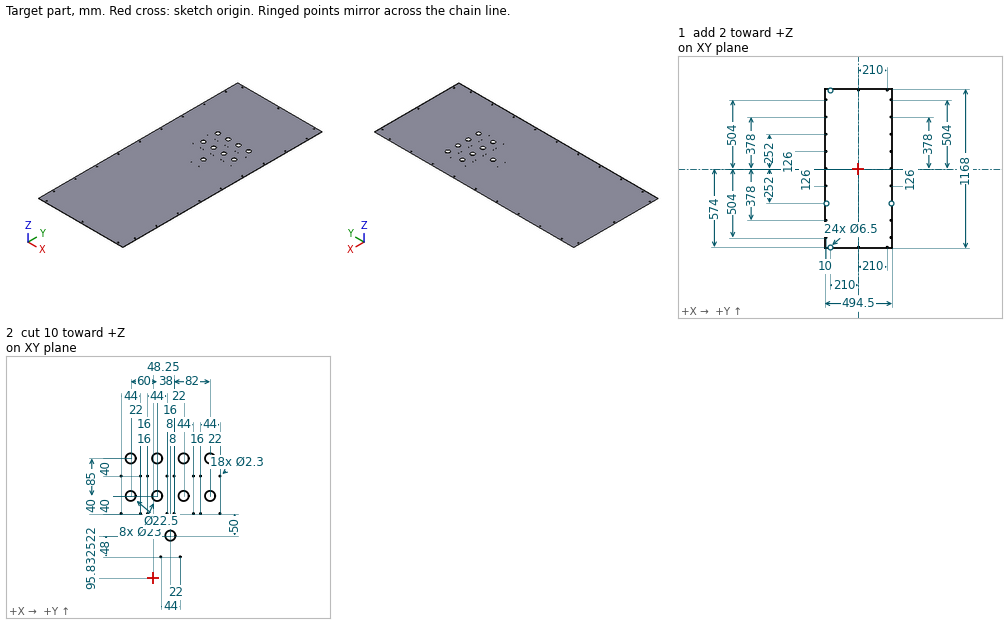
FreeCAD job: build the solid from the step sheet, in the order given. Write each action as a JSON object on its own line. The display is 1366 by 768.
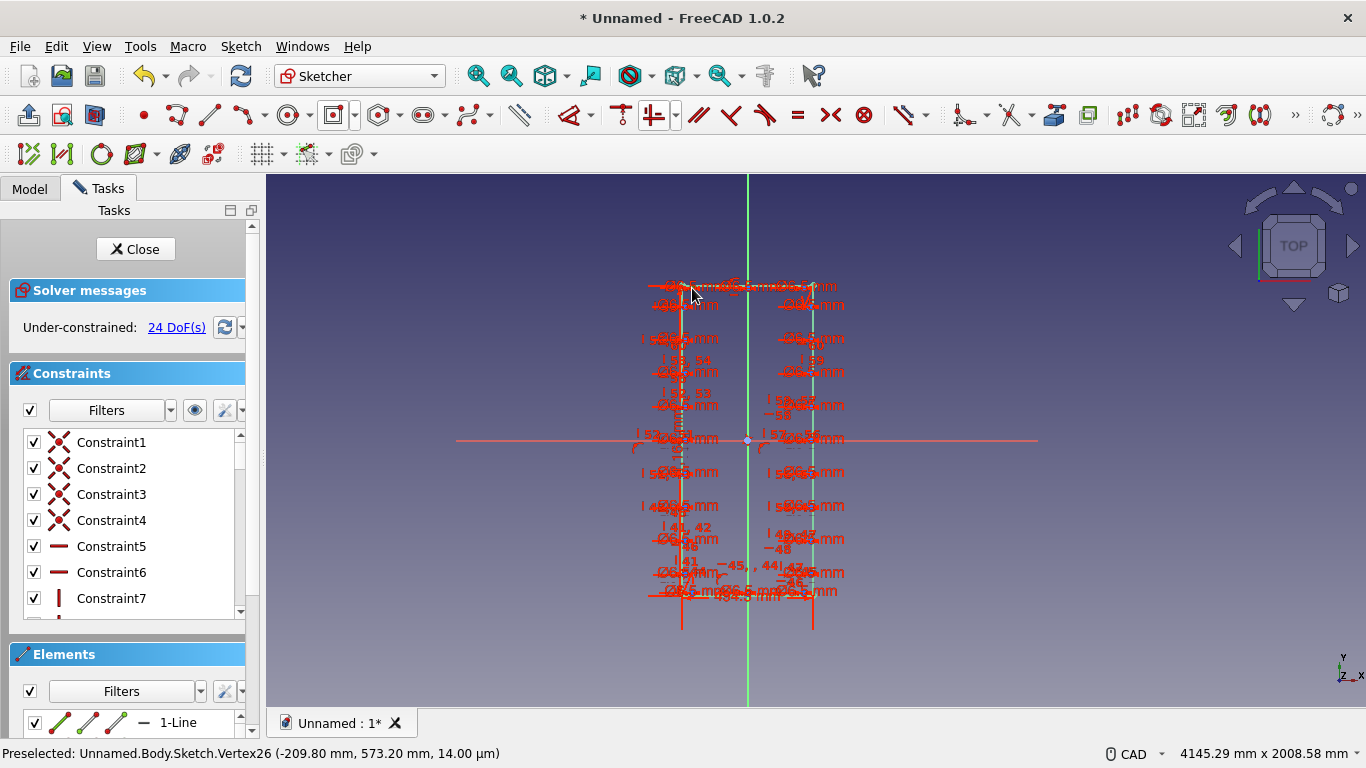
{"action": "left_click", "coordinate": [748, 288]}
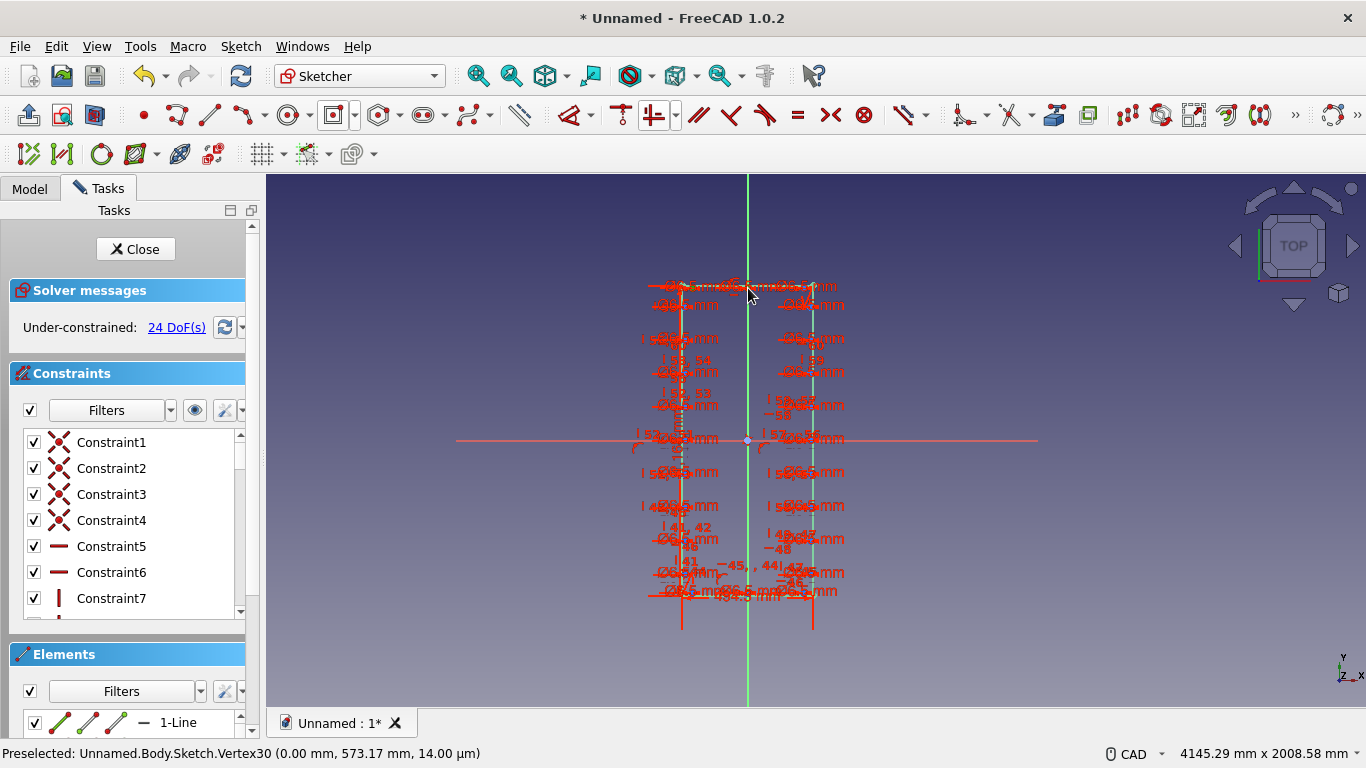
{"action": "left_click", "coordinate": [676, 116]}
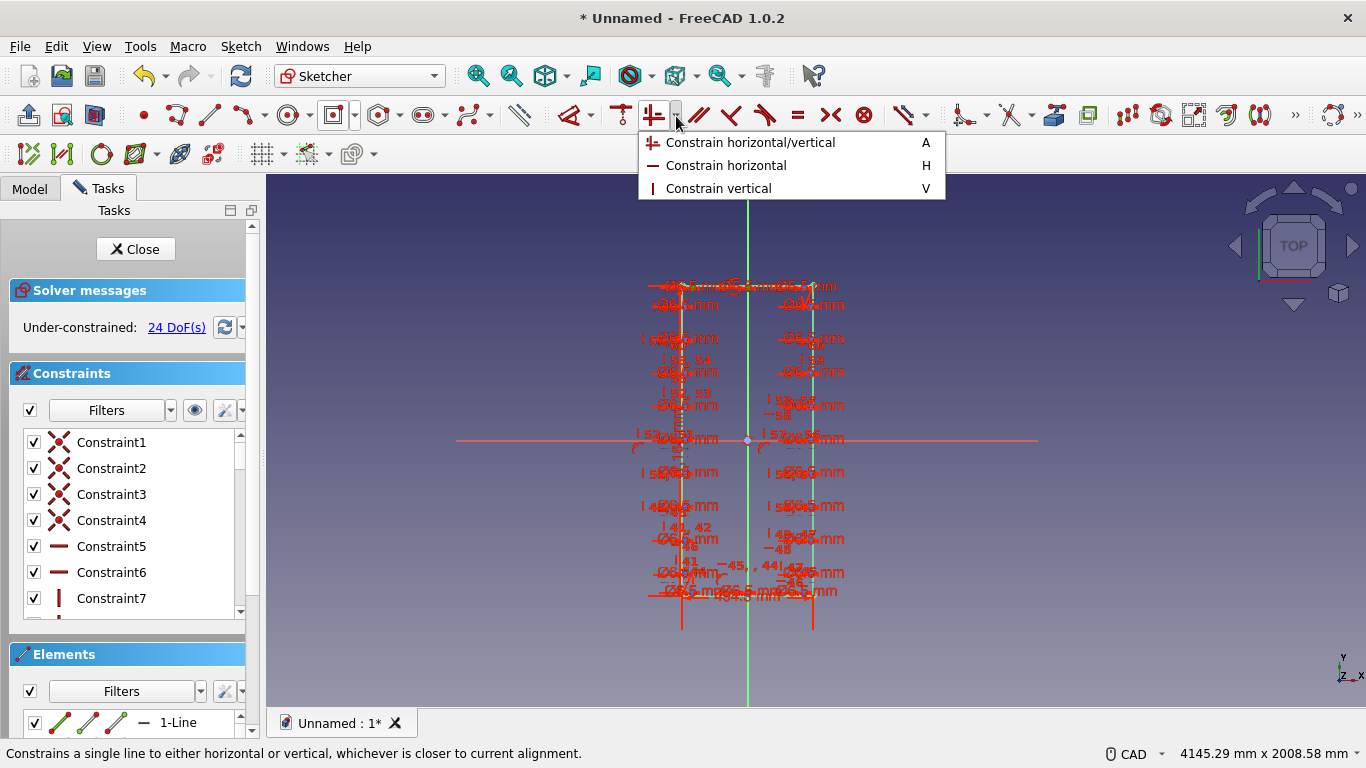
{"action": "left_click", "coordinate": [792, 166]}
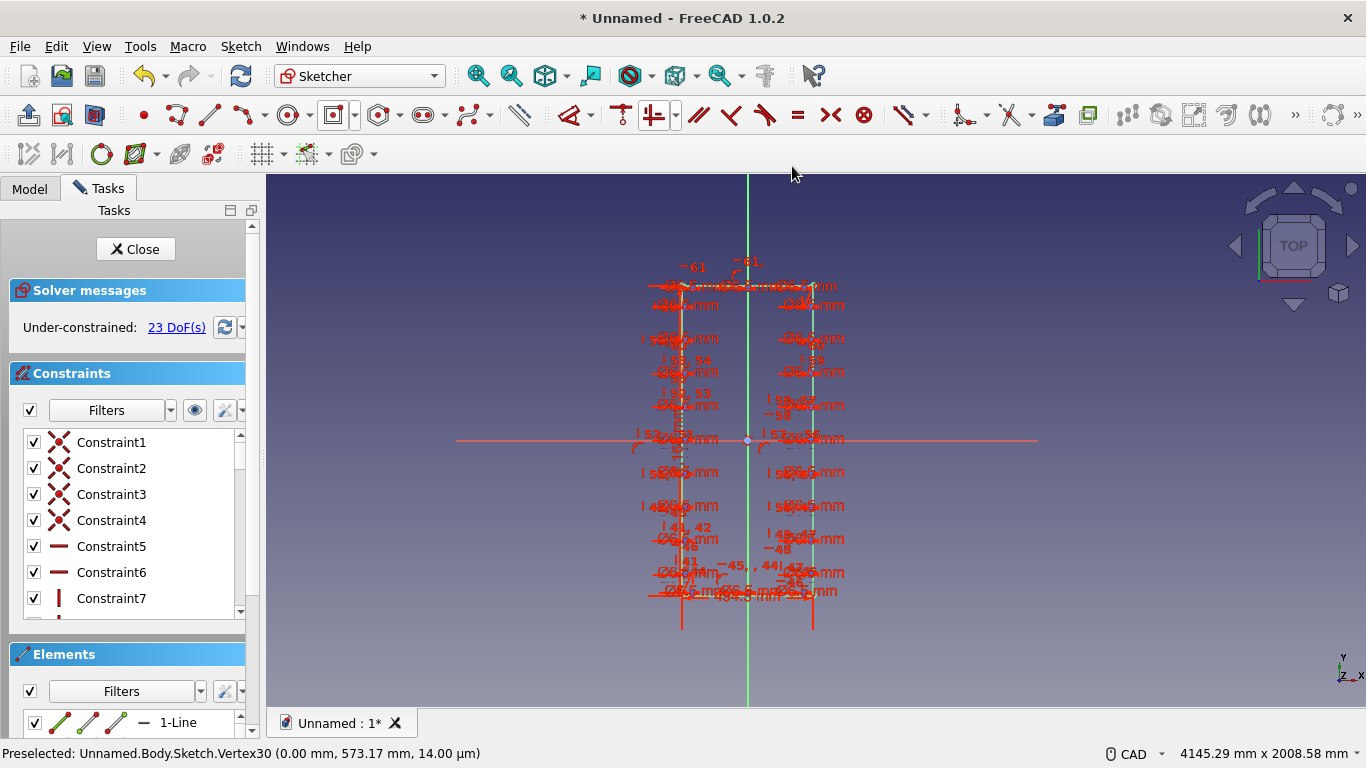
{"action": "left_click", "coordinate": [811, 374]}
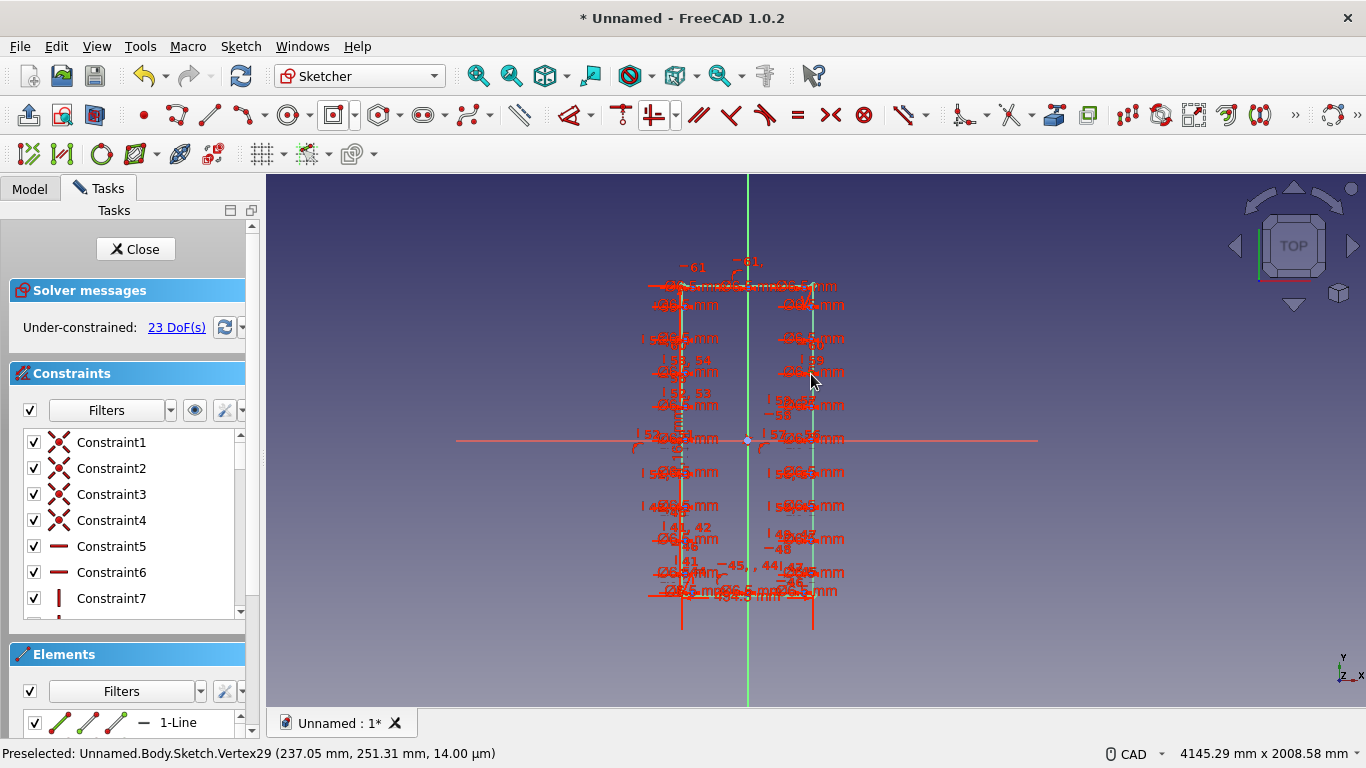
{"action": "scroll", "coordinate": [811, 340], "scroll_direction": "up", "scroll_amount": 4}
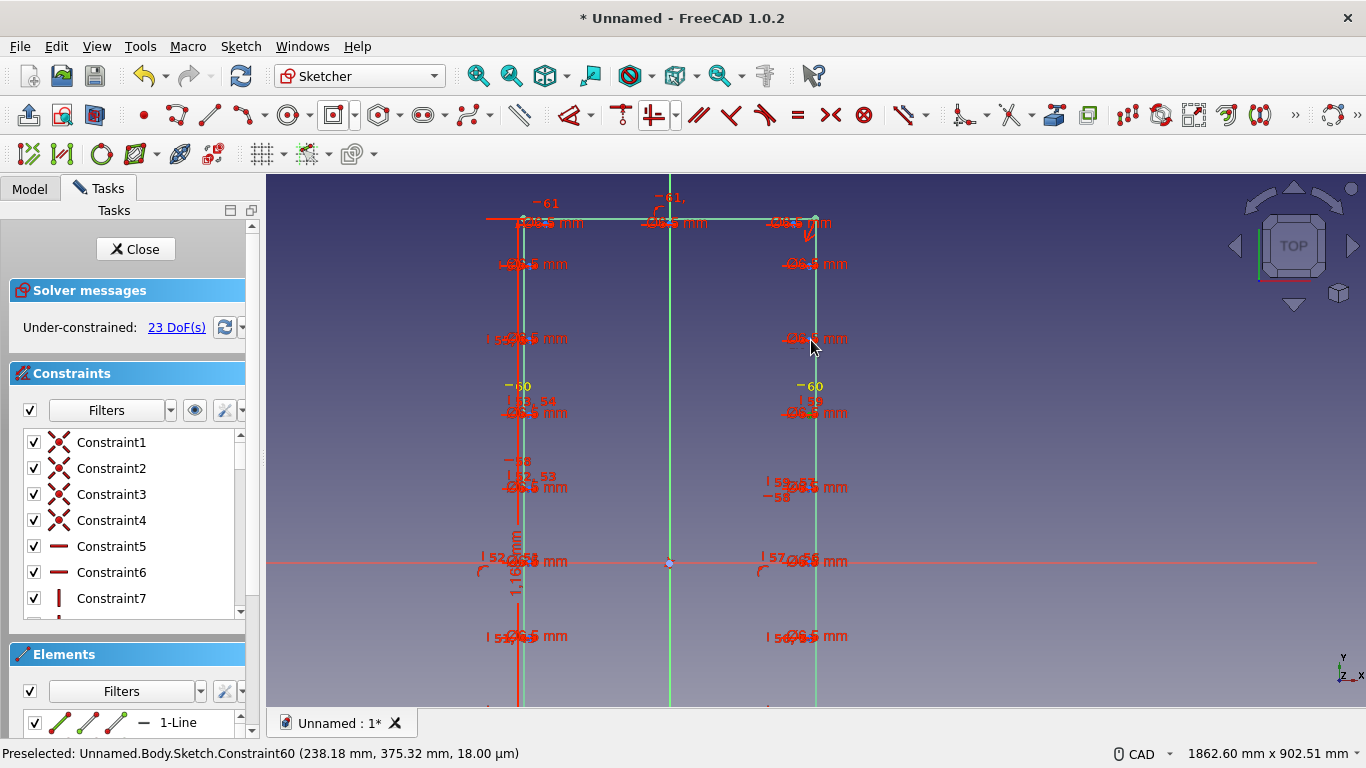
{"action": "left_click", "coordinate": [810, 341]}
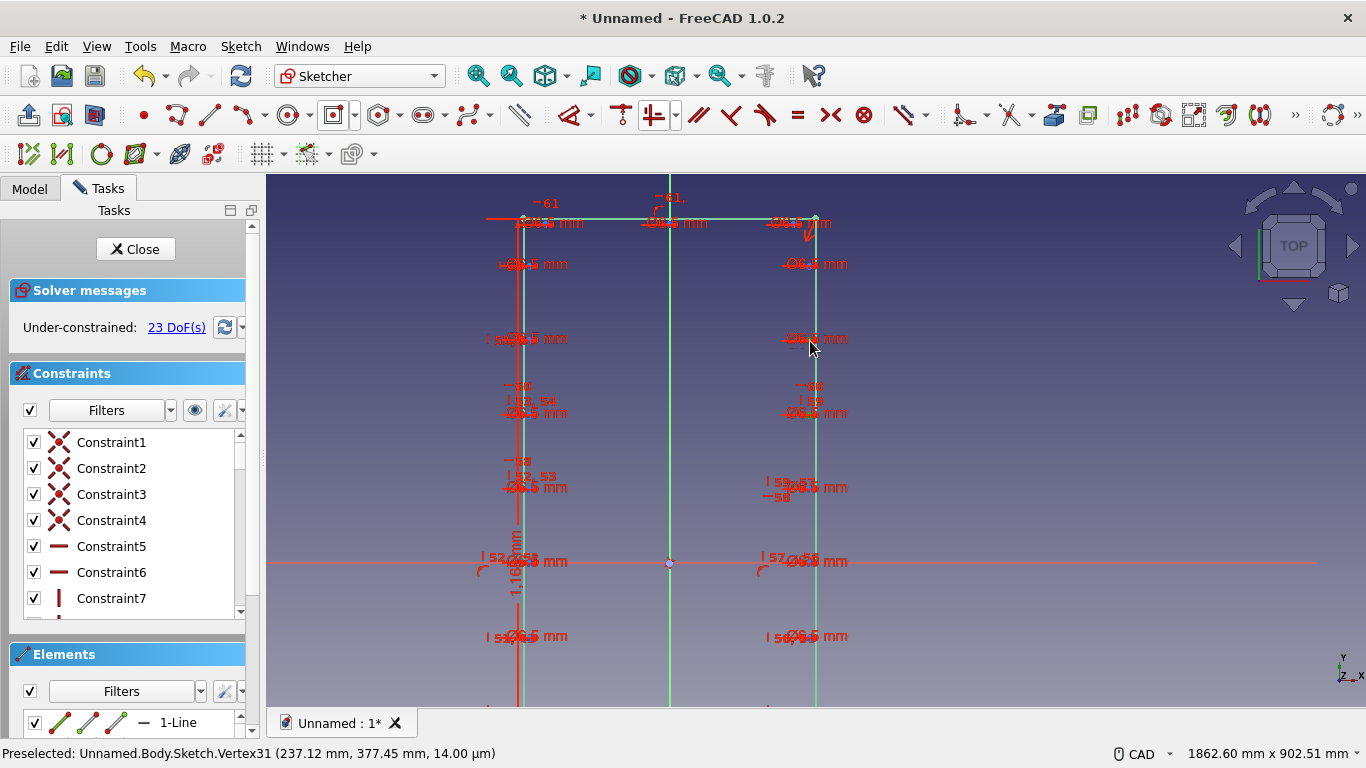
{"action": "left_click", "coordinate": [676, 116]}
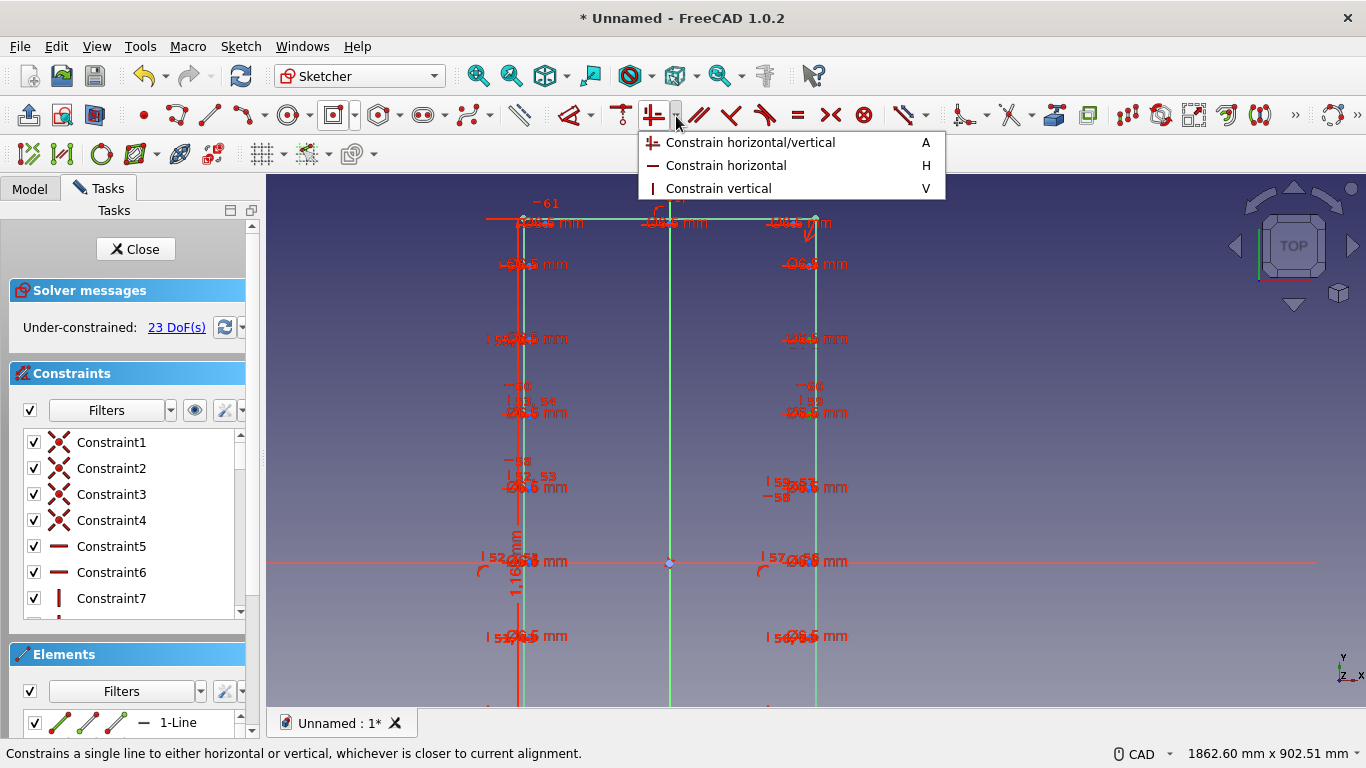
{"action": "left_click", "coordinate": [792, 188]}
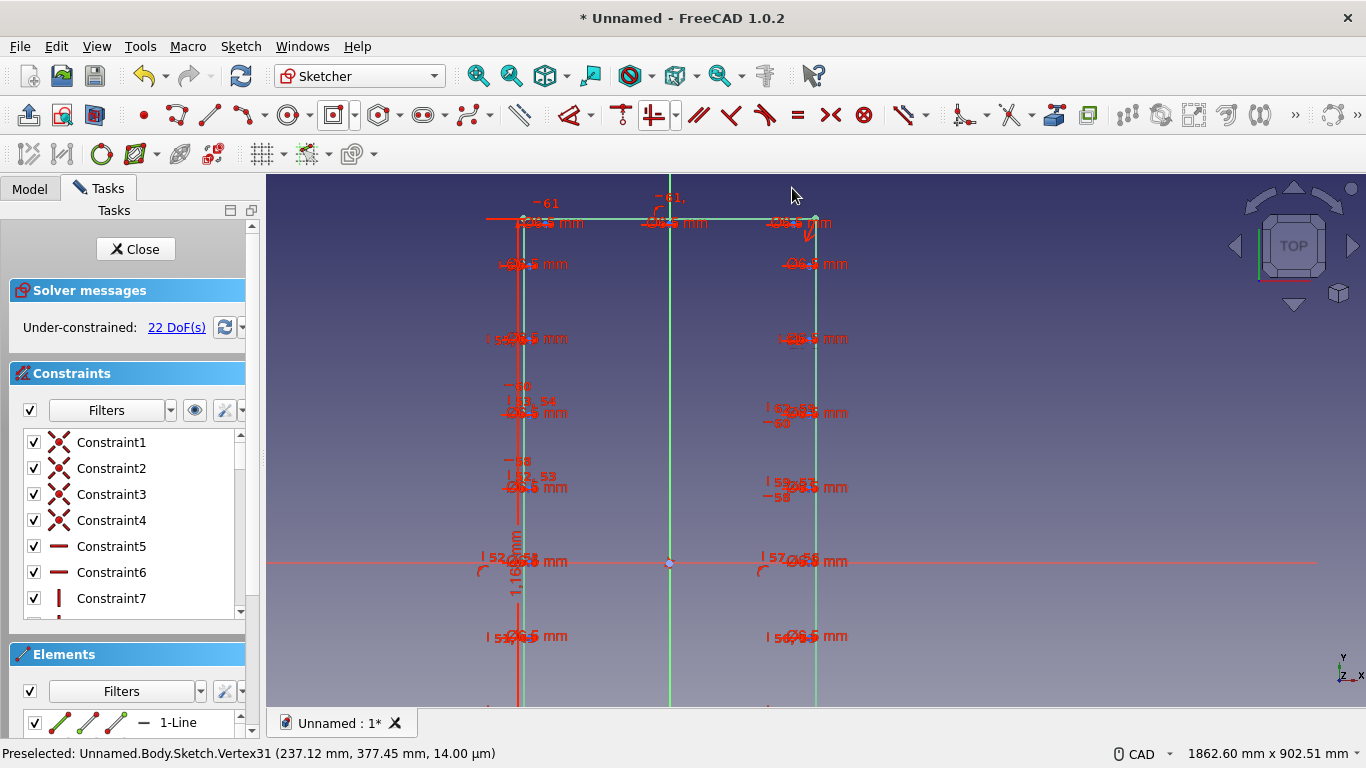
{"action": "left_click", "coordinate": [810, 341]}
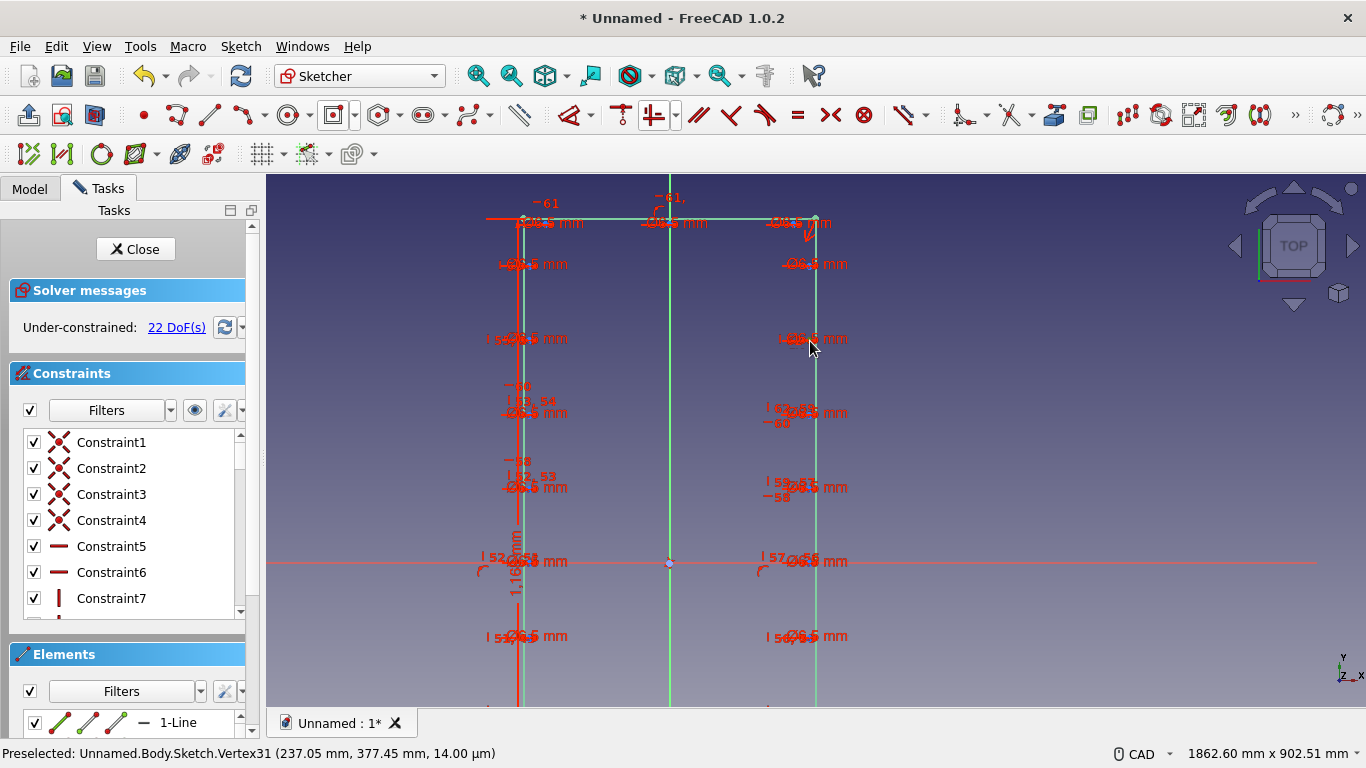
{"action": "left_click", "coordinate": [810, 266]}